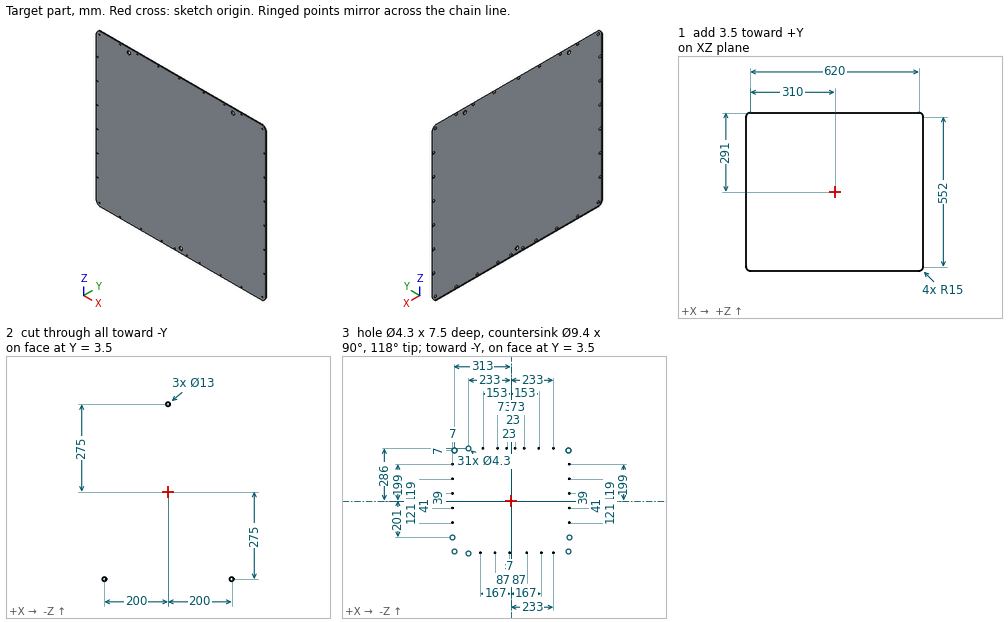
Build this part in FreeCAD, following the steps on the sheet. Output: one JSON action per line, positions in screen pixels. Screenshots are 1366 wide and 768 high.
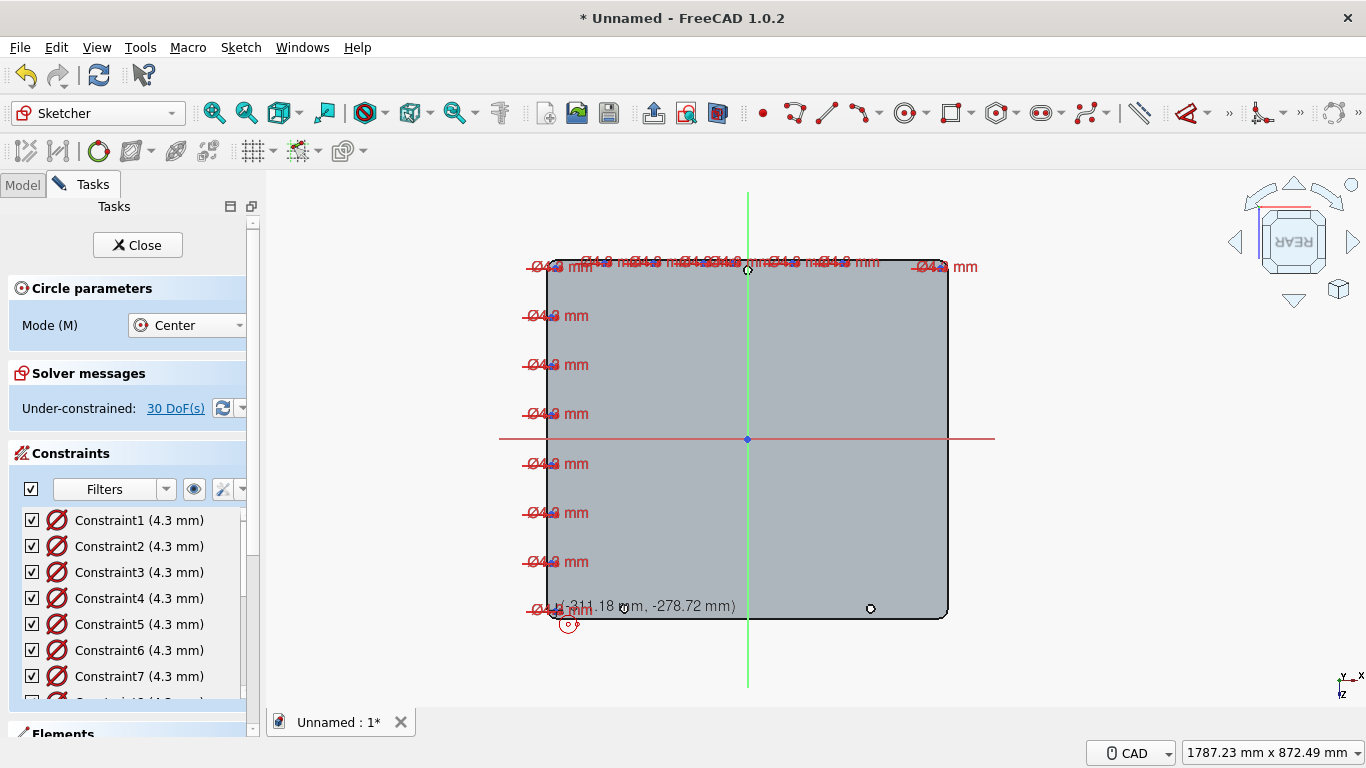
{"action": "scroll", "coordinate": [604, 615], "scroll_direction": "up", "scroll_amount": 15}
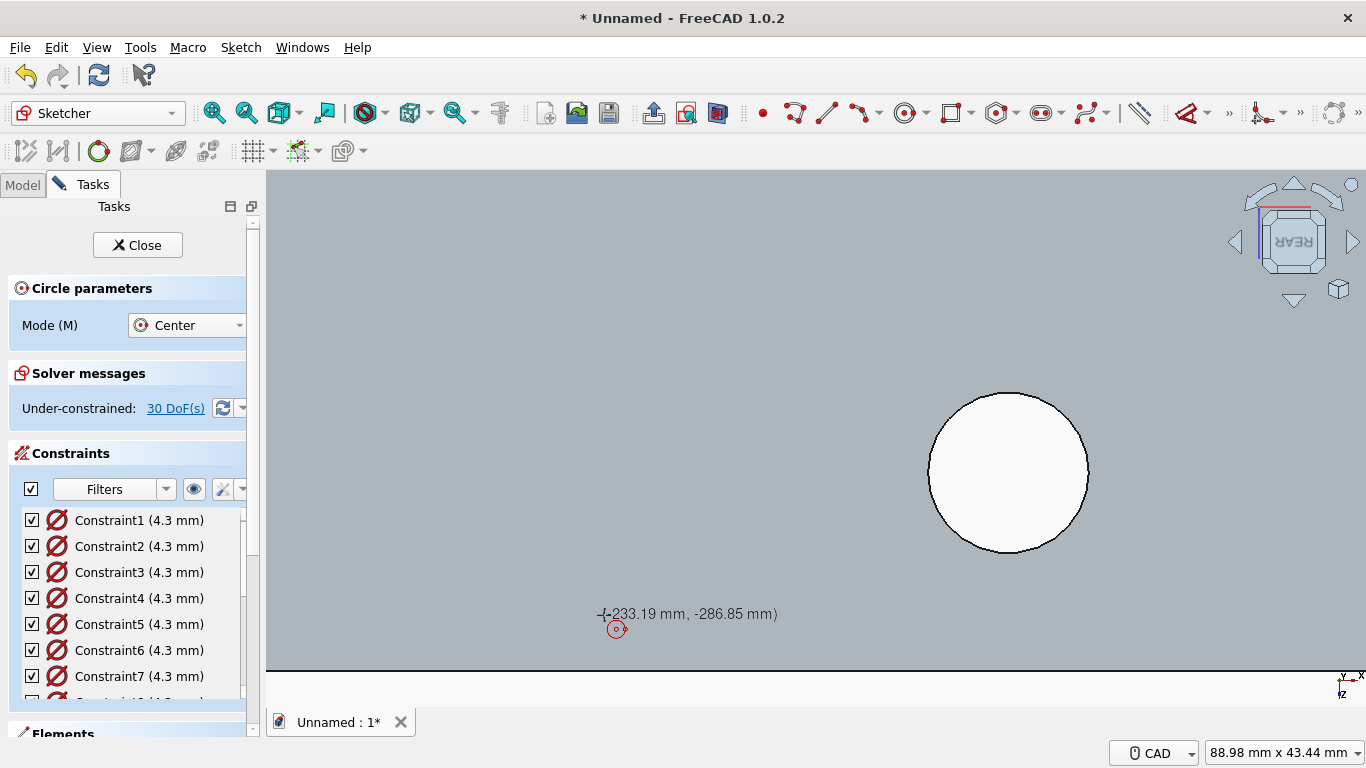
{"action": "scroll", "coordinate": [604, 615], "scroll_direction": "down", "scroll_amount": 15}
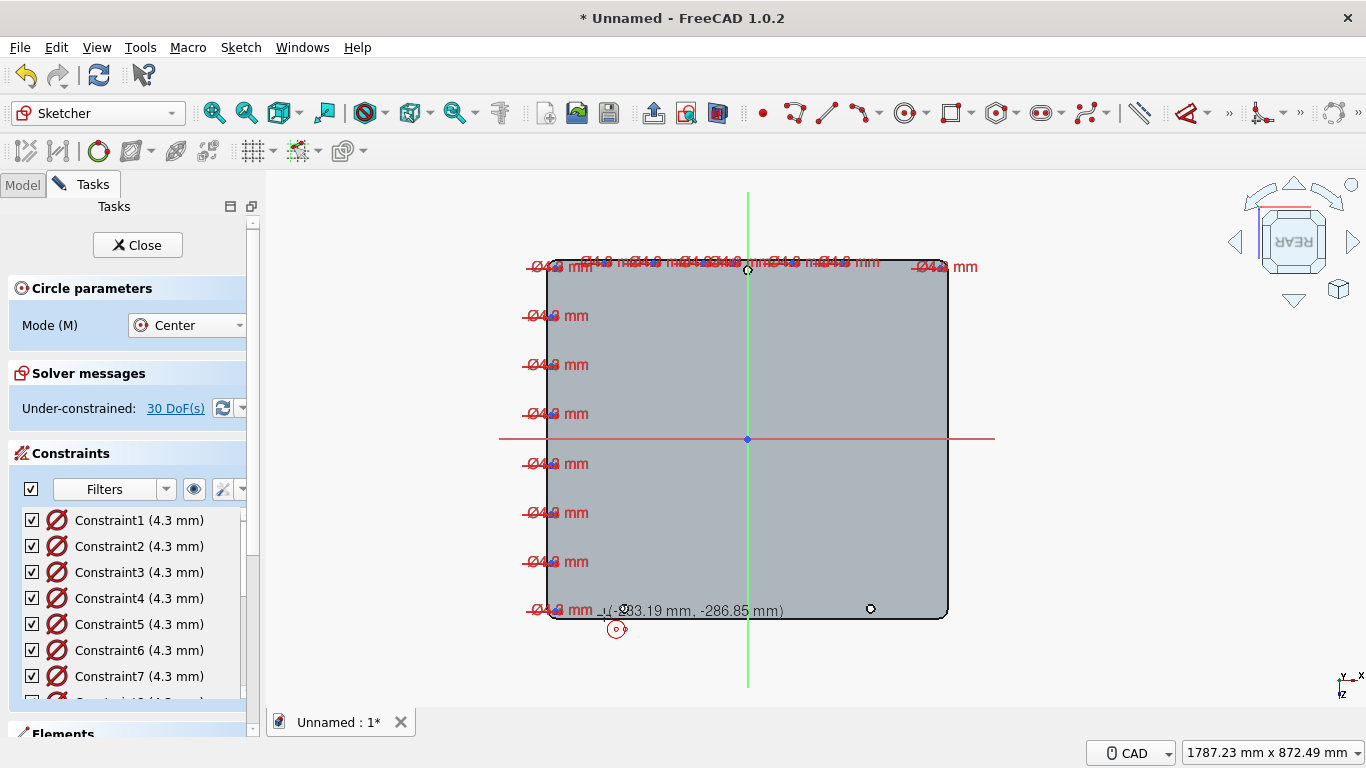
{"action": "left_click", "coordinate": [604, 615]}
{"action": "mouse_move", "coordinate": [605, 615]}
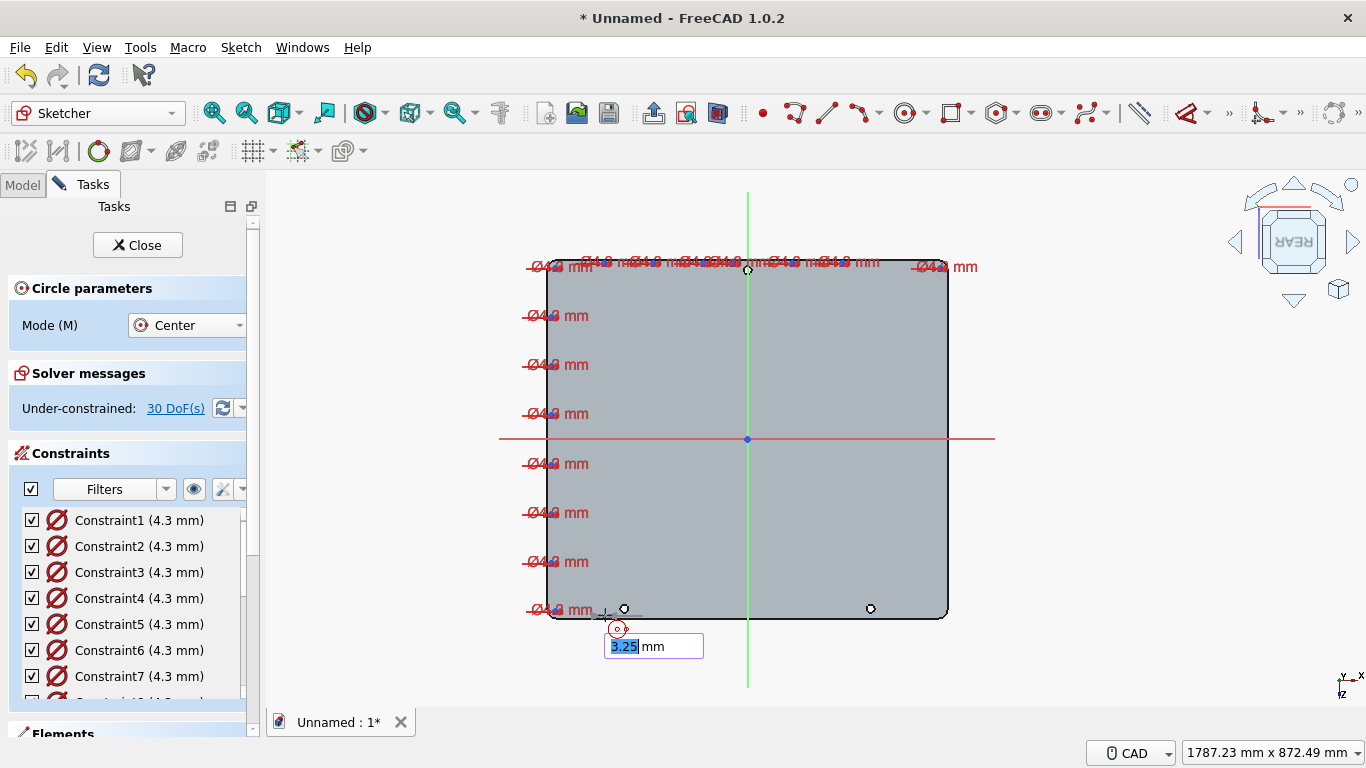
{"action": "type", "text": "4.3"}
{"action": "key", "text": "Return"}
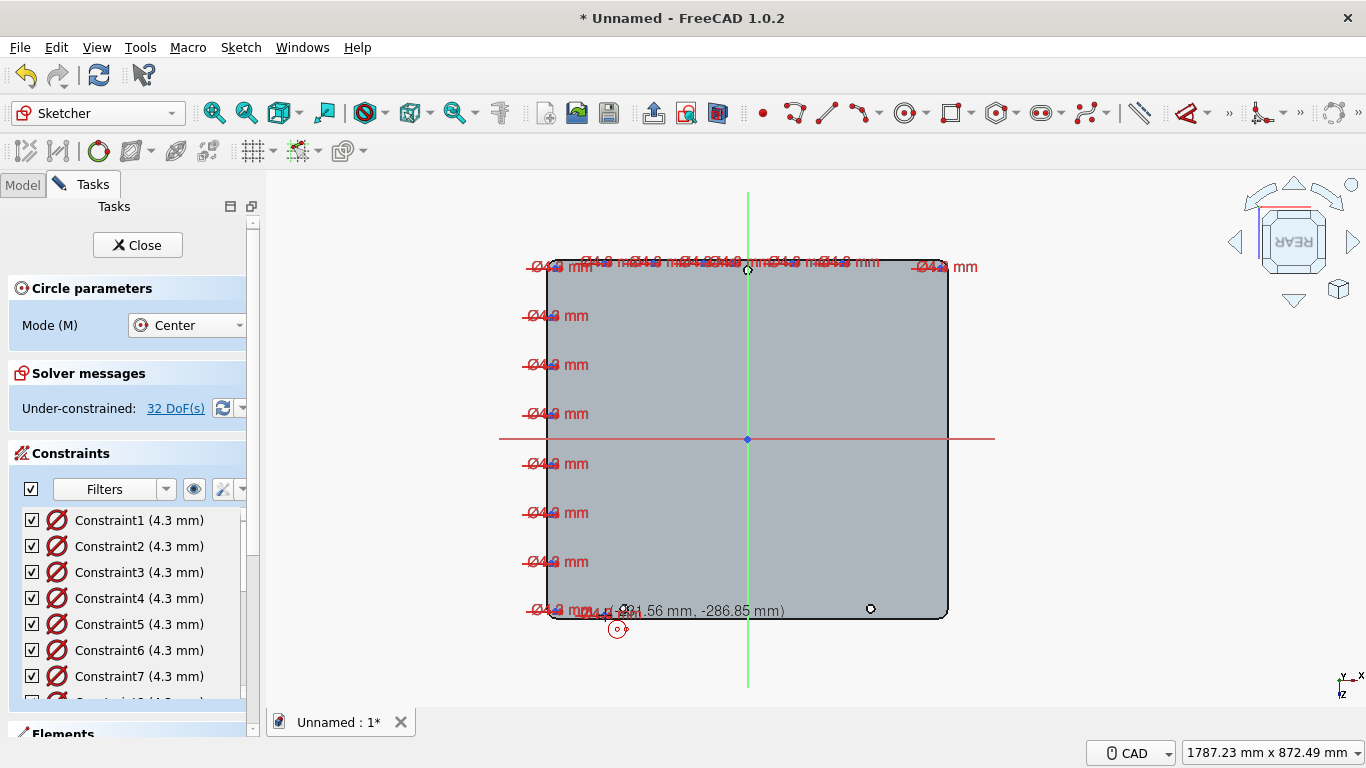
{"action": "scroll", "coordinate": [645, 615], "scroll_direction": "up", "scroll_amount": 15}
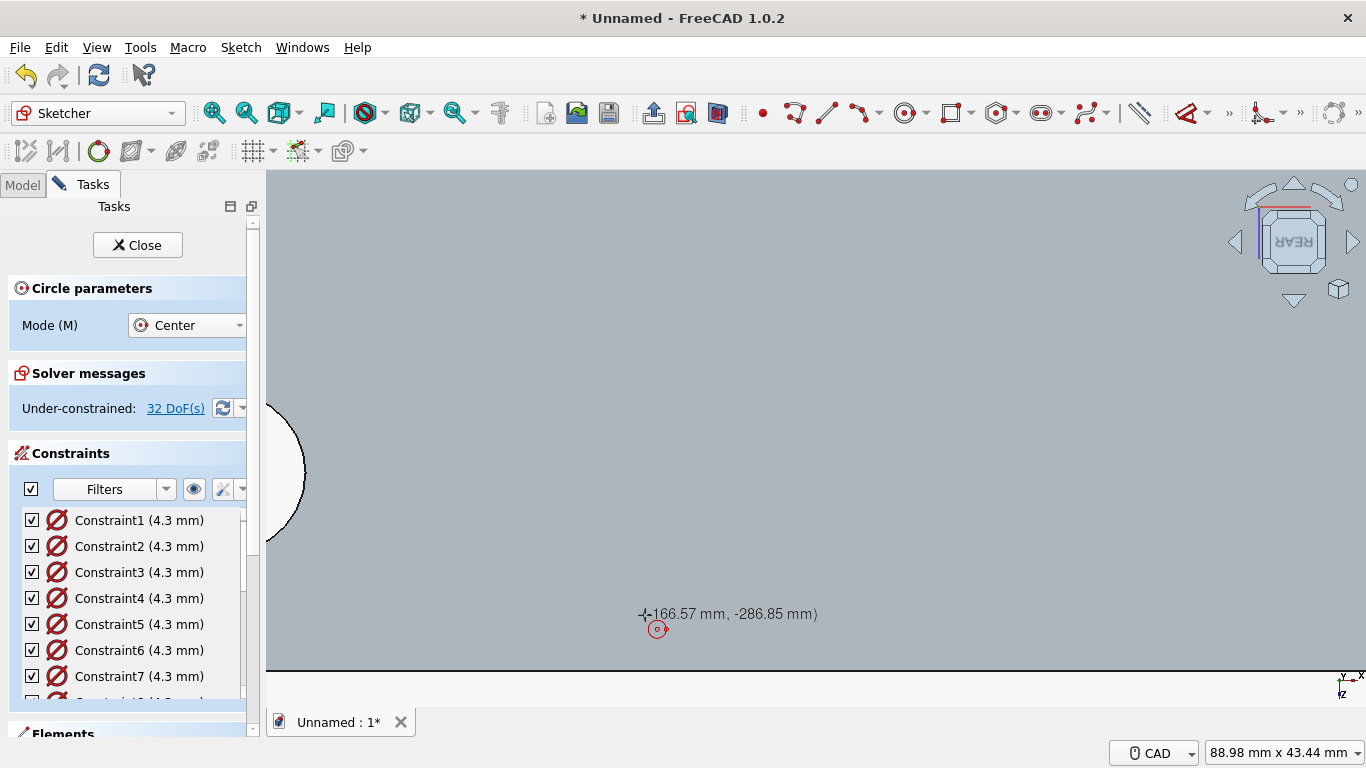
{"action": "scroll", "coordinate": [645, 615], "scroll_direction": "down", "scroll_amount": 15}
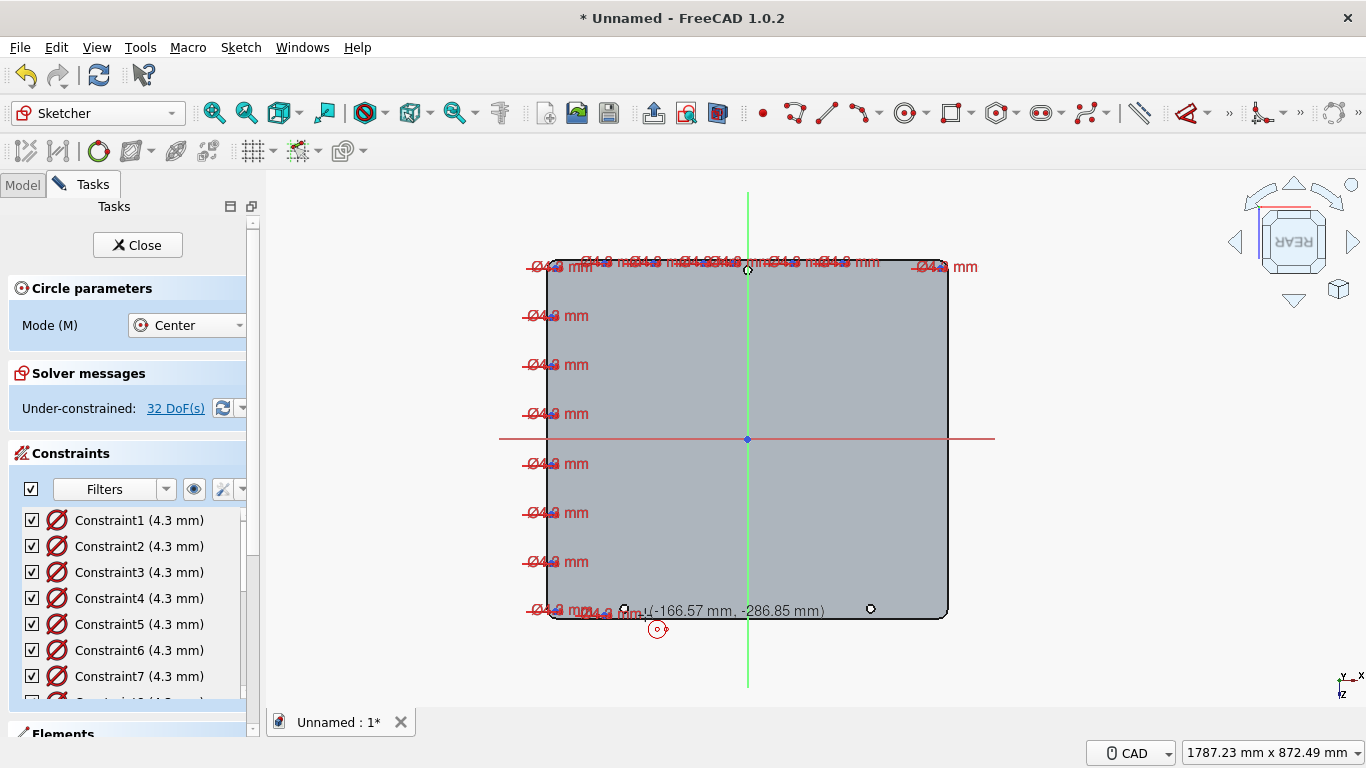
{"action": "left_click", "coordinate": [645, 615]}
{"action": "mouse_move", "coordinate": [646, 615]}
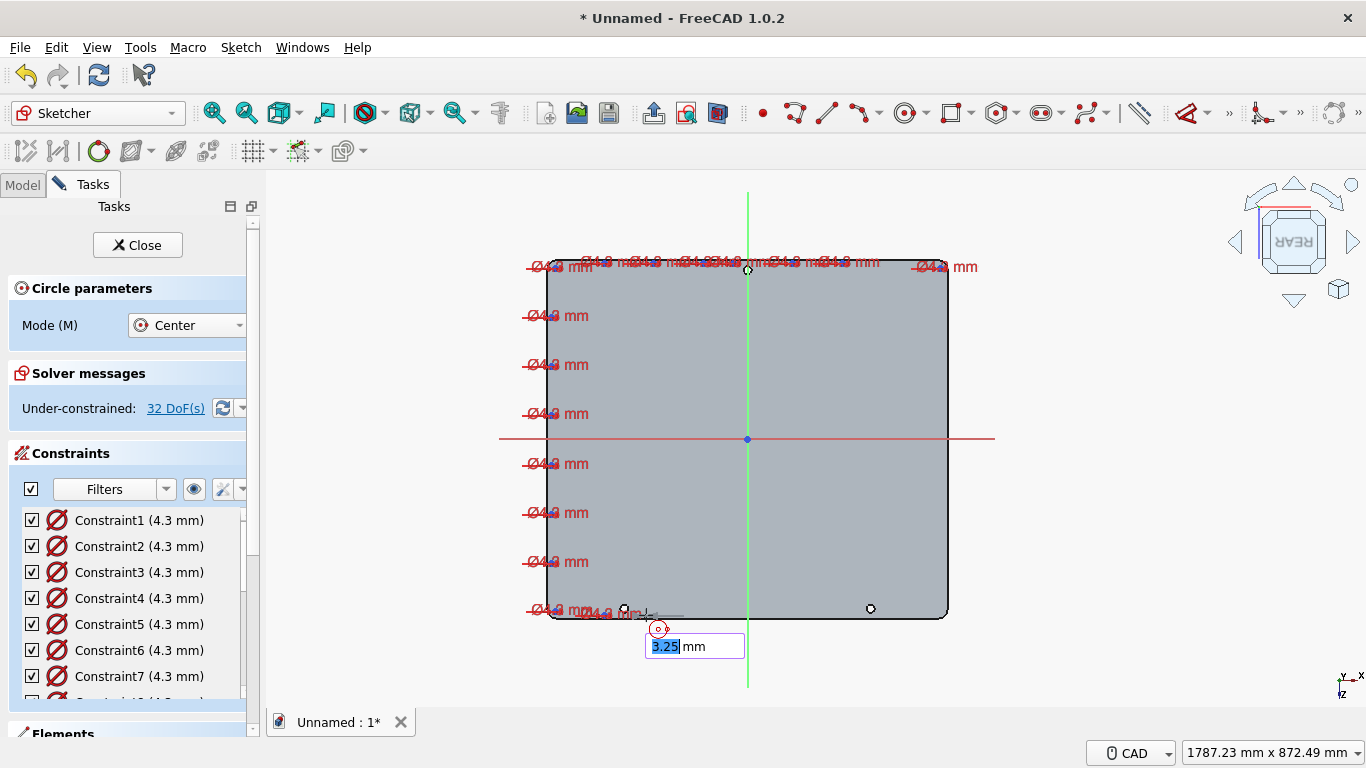
{"action": "type", "text": "4.3"}
{"action": "key", "text": "Return"}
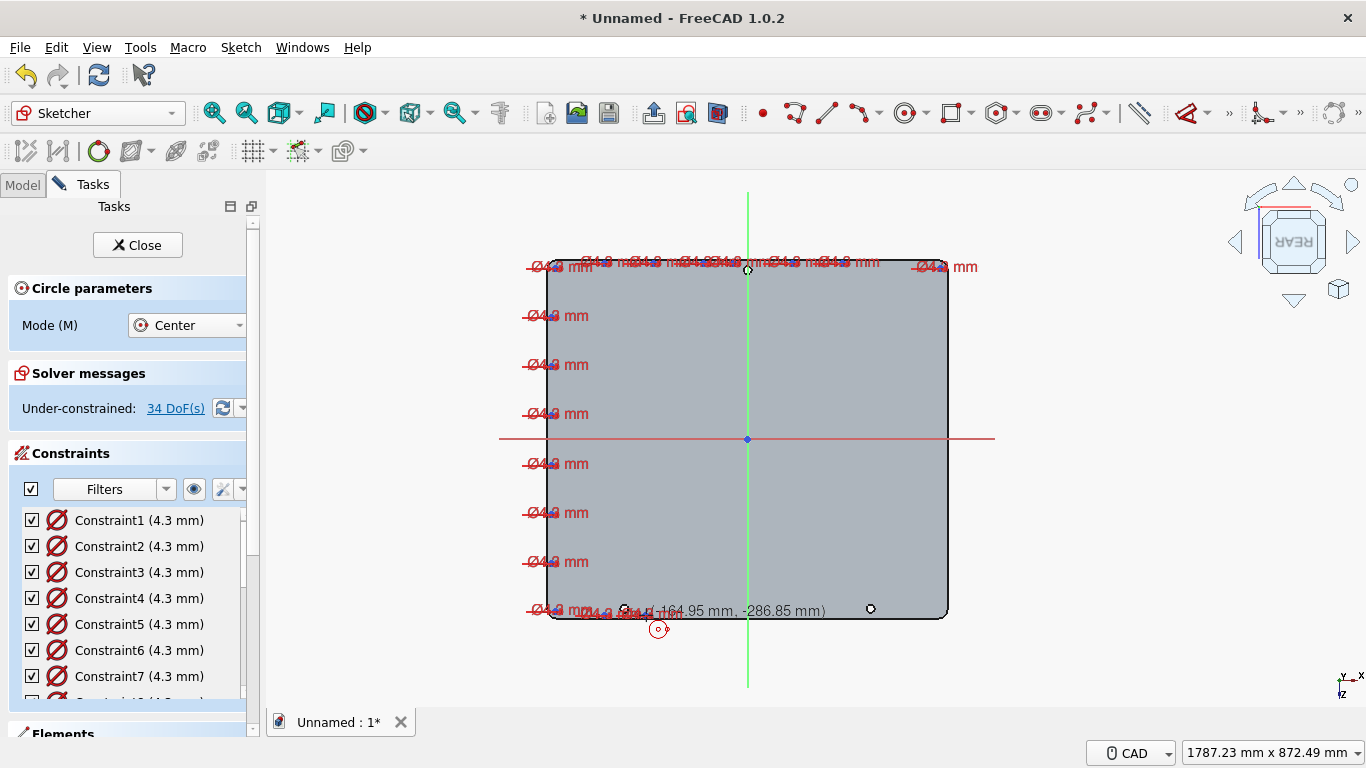
{"action": "scroll", "coordinate": [694, 615], "scroll_direction": "up", "scroll_amount": 15}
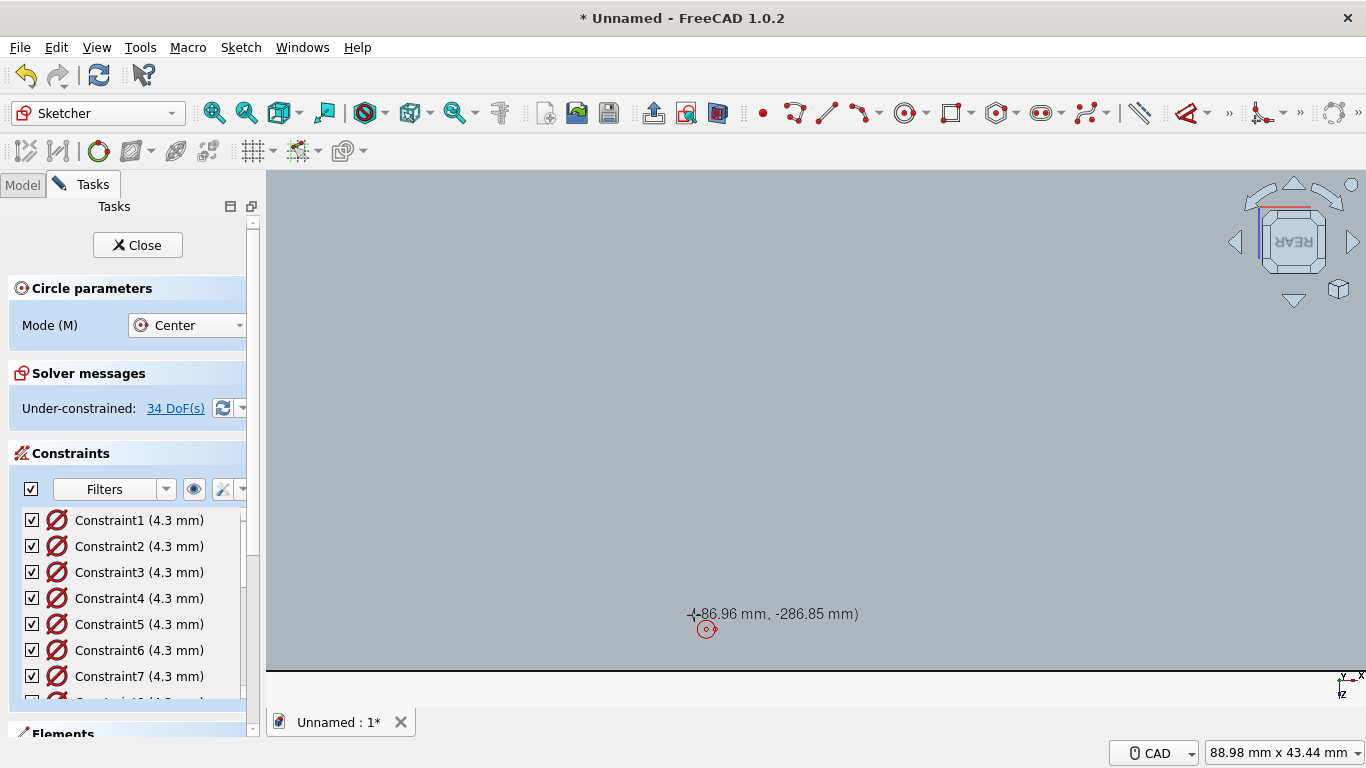
{"action": "scroll", "coordinate": [694, 615], "scroll_direction": "down", "scroll_amount": 15}